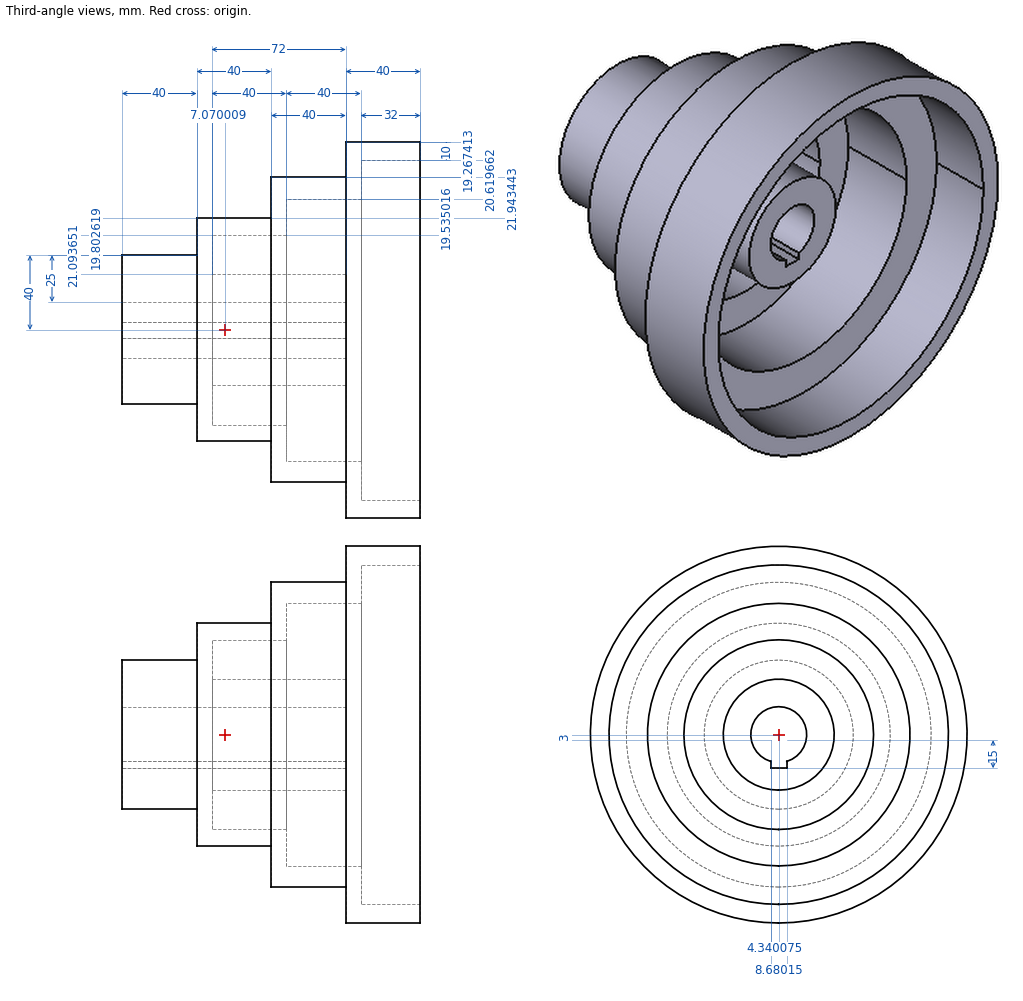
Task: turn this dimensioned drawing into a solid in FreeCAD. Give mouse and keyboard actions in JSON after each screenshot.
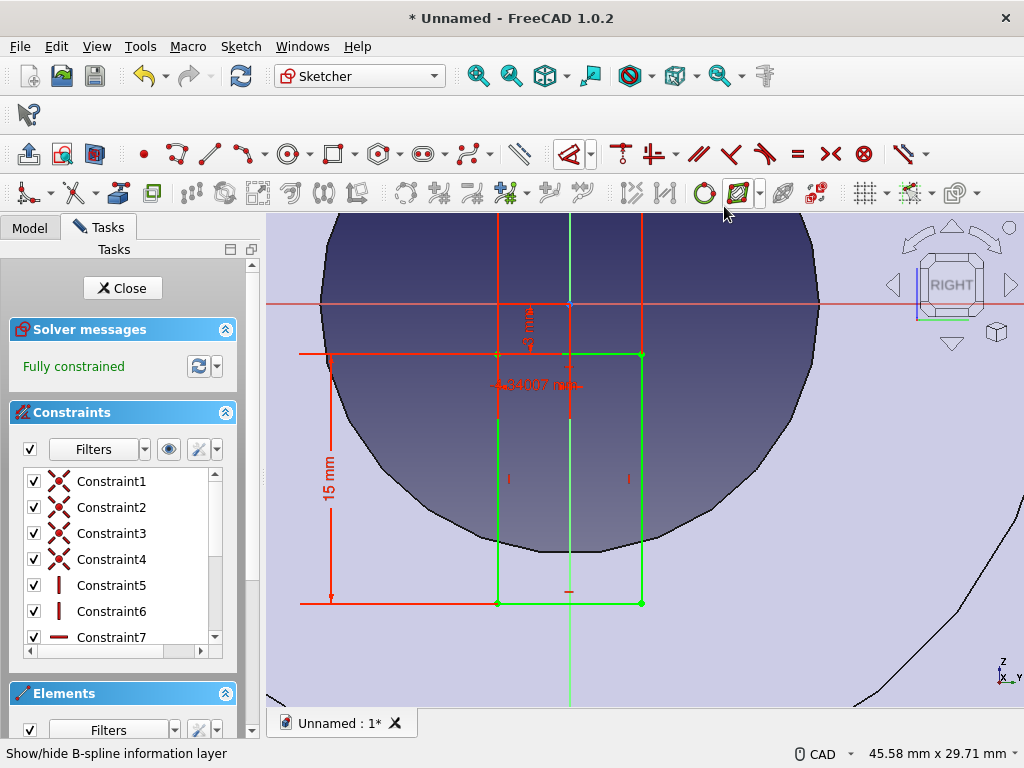
{"action": "left_click", "coordinate": [123, 288]}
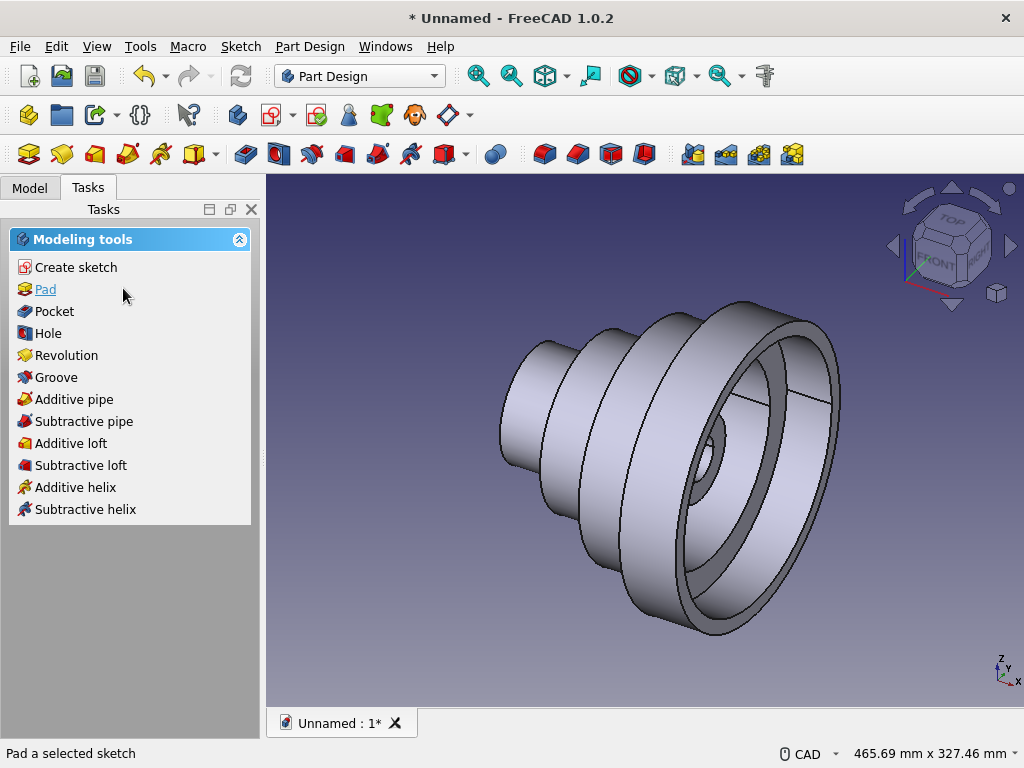
{"action": "left_click", "coordinate": [246, 154]}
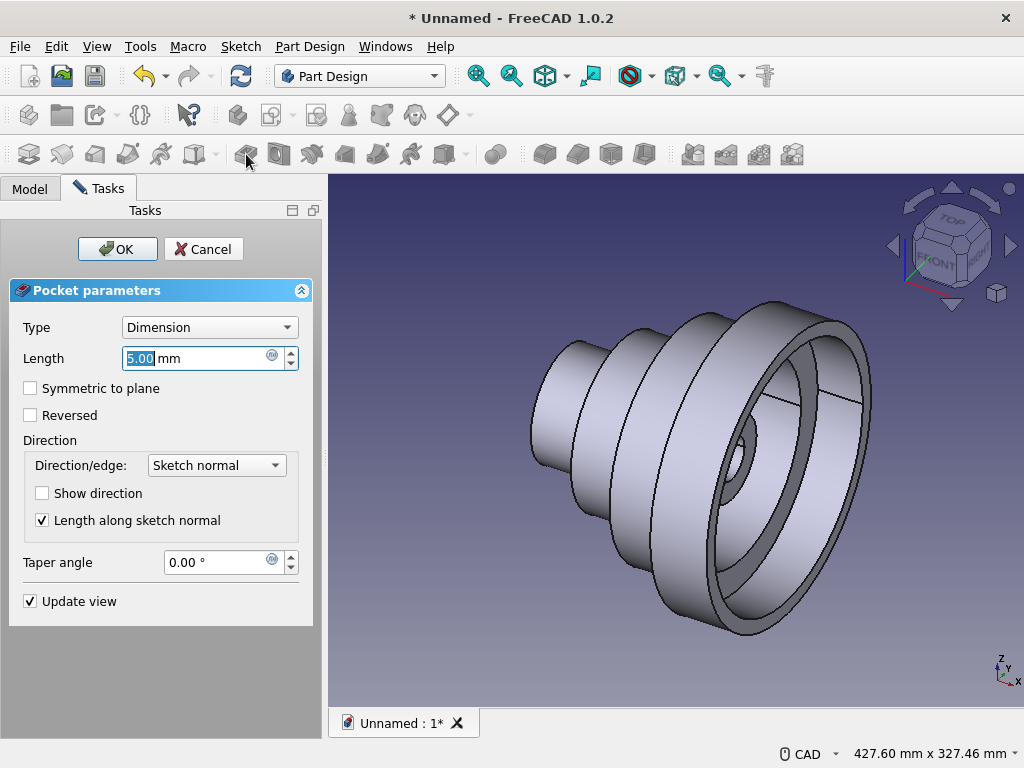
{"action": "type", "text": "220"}
{"action": "key", "text": "Tab"}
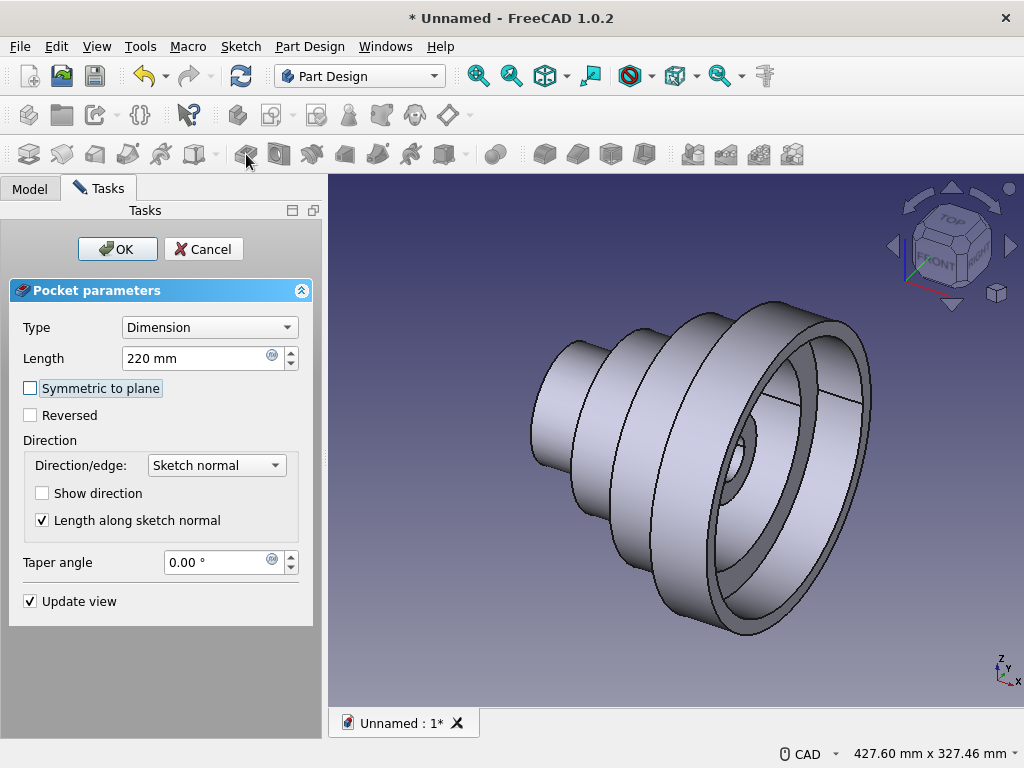
{"action": "left_click", "coordinate": [31, 388]}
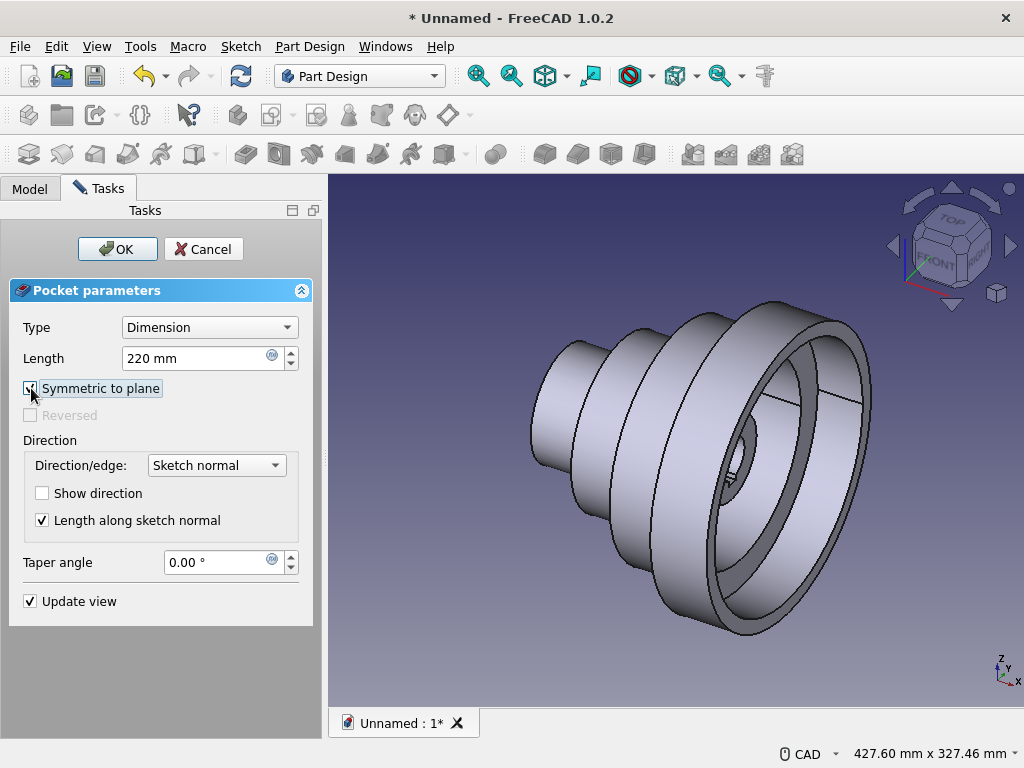
{"action": "left_click", "coordinate": [118, 249]}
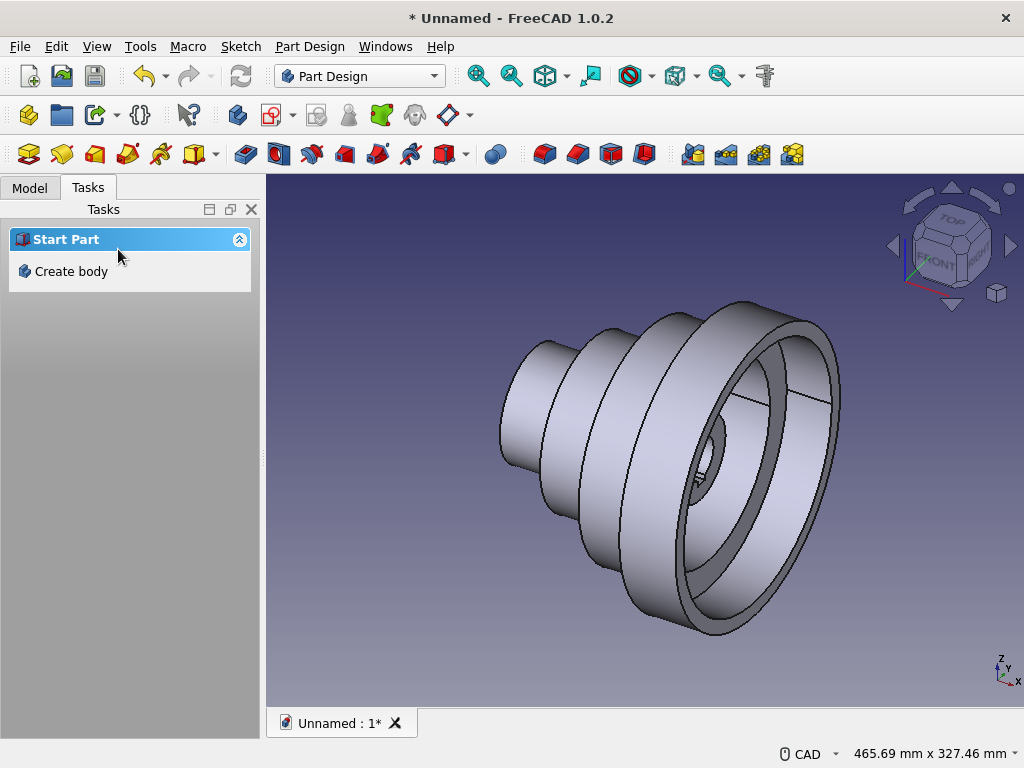
{"action": "key", "text": "0"}